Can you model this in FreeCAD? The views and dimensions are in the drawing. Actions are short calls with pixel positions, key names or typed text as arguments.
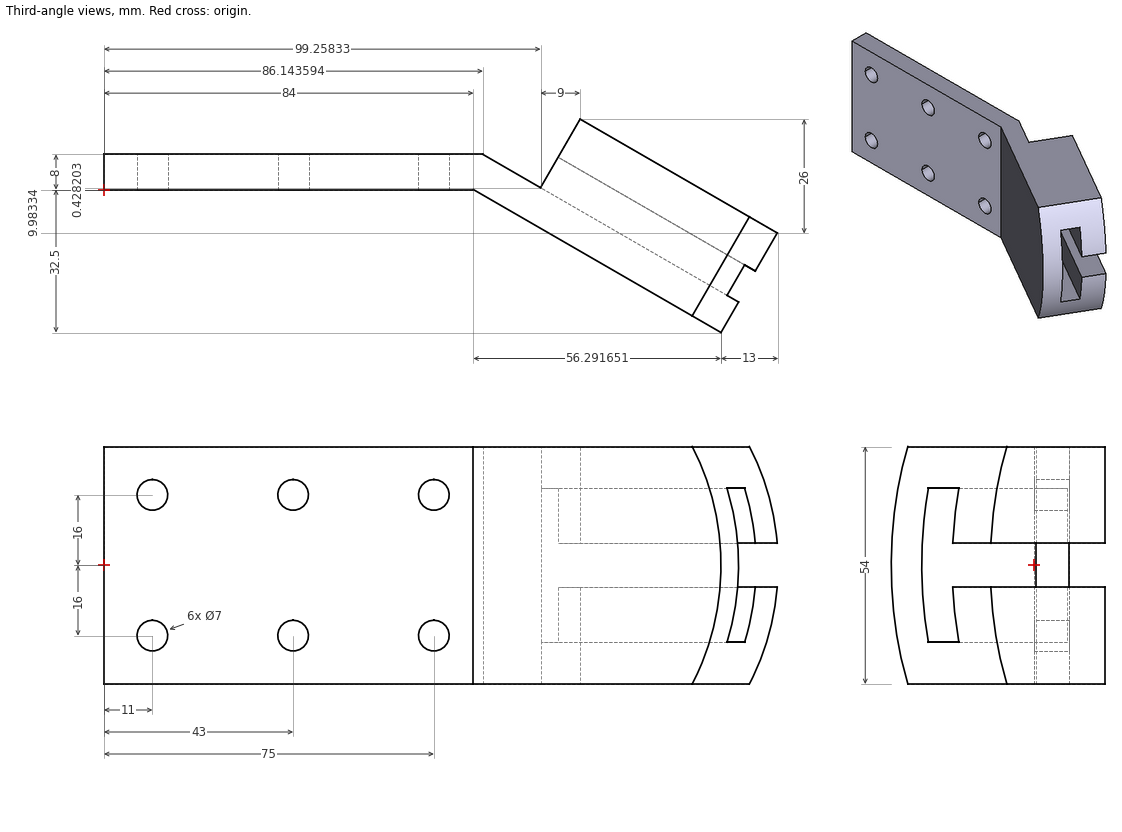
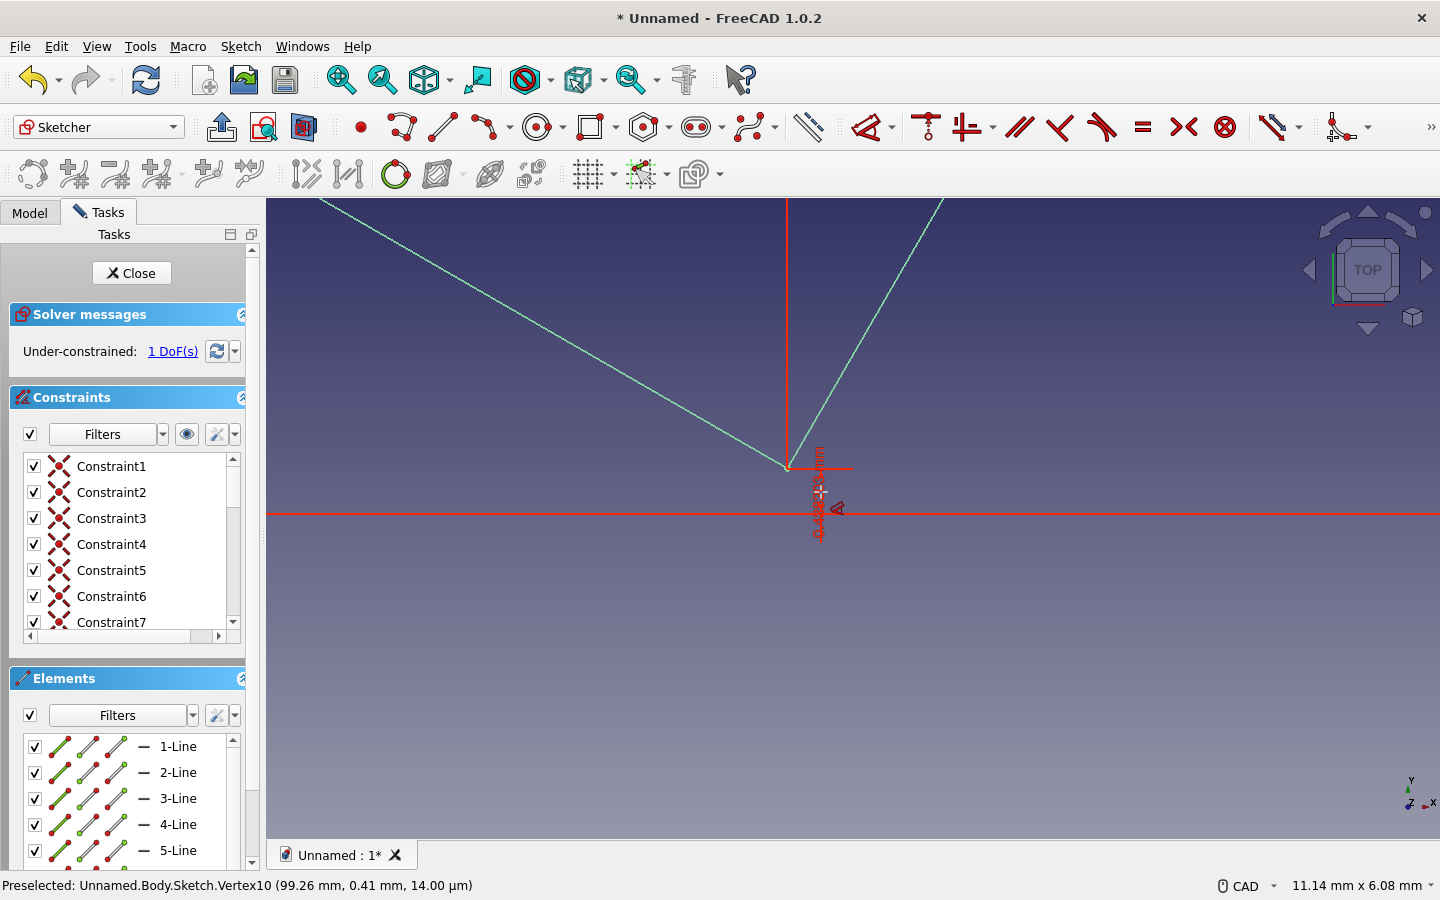
scroll(909, 473, down, 15)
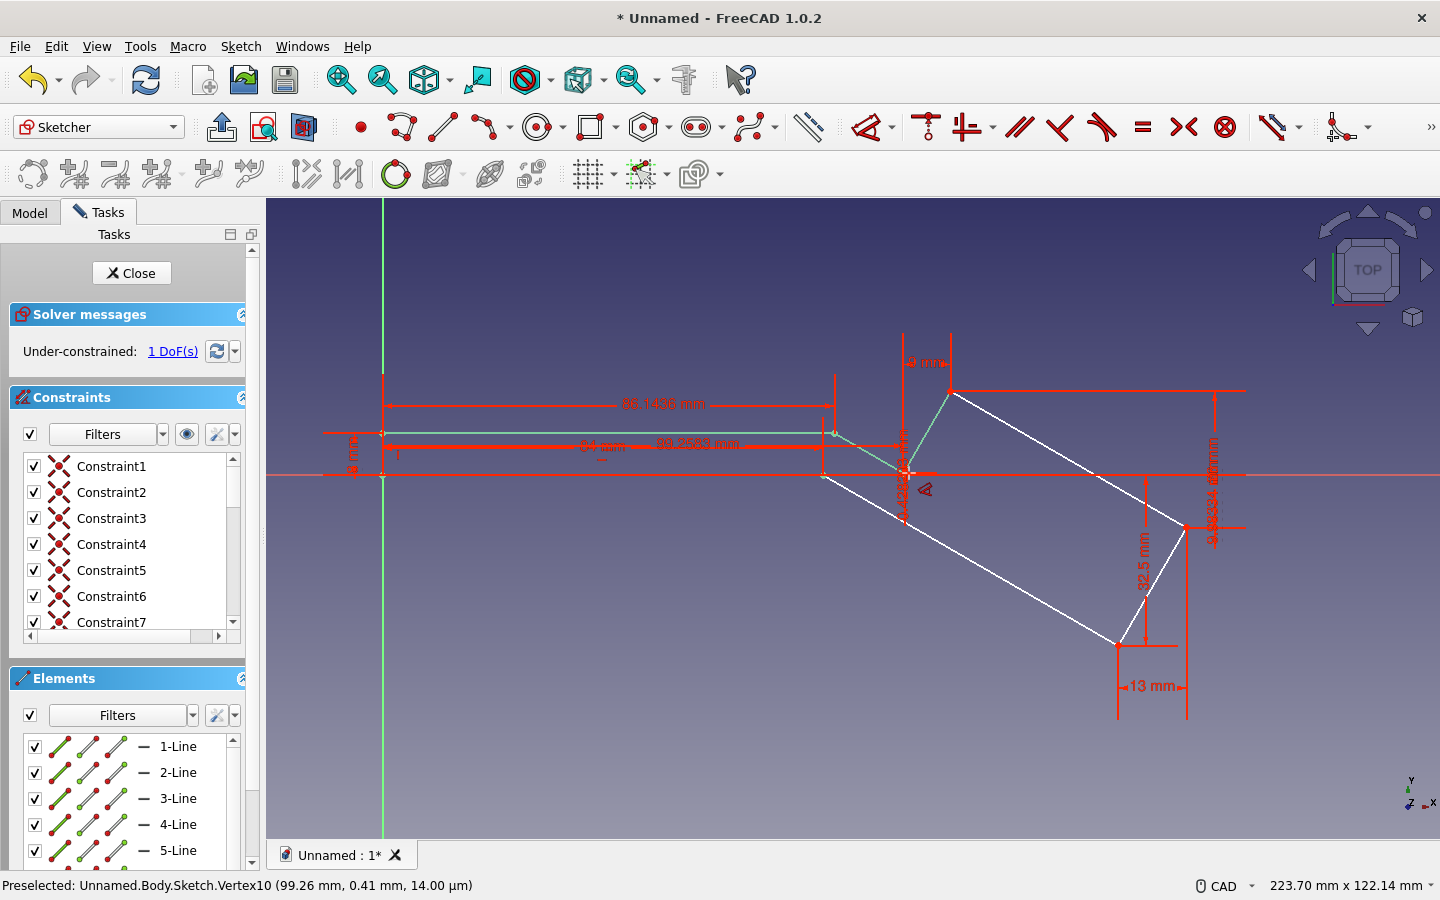
click(912, 527)
click(971, 680)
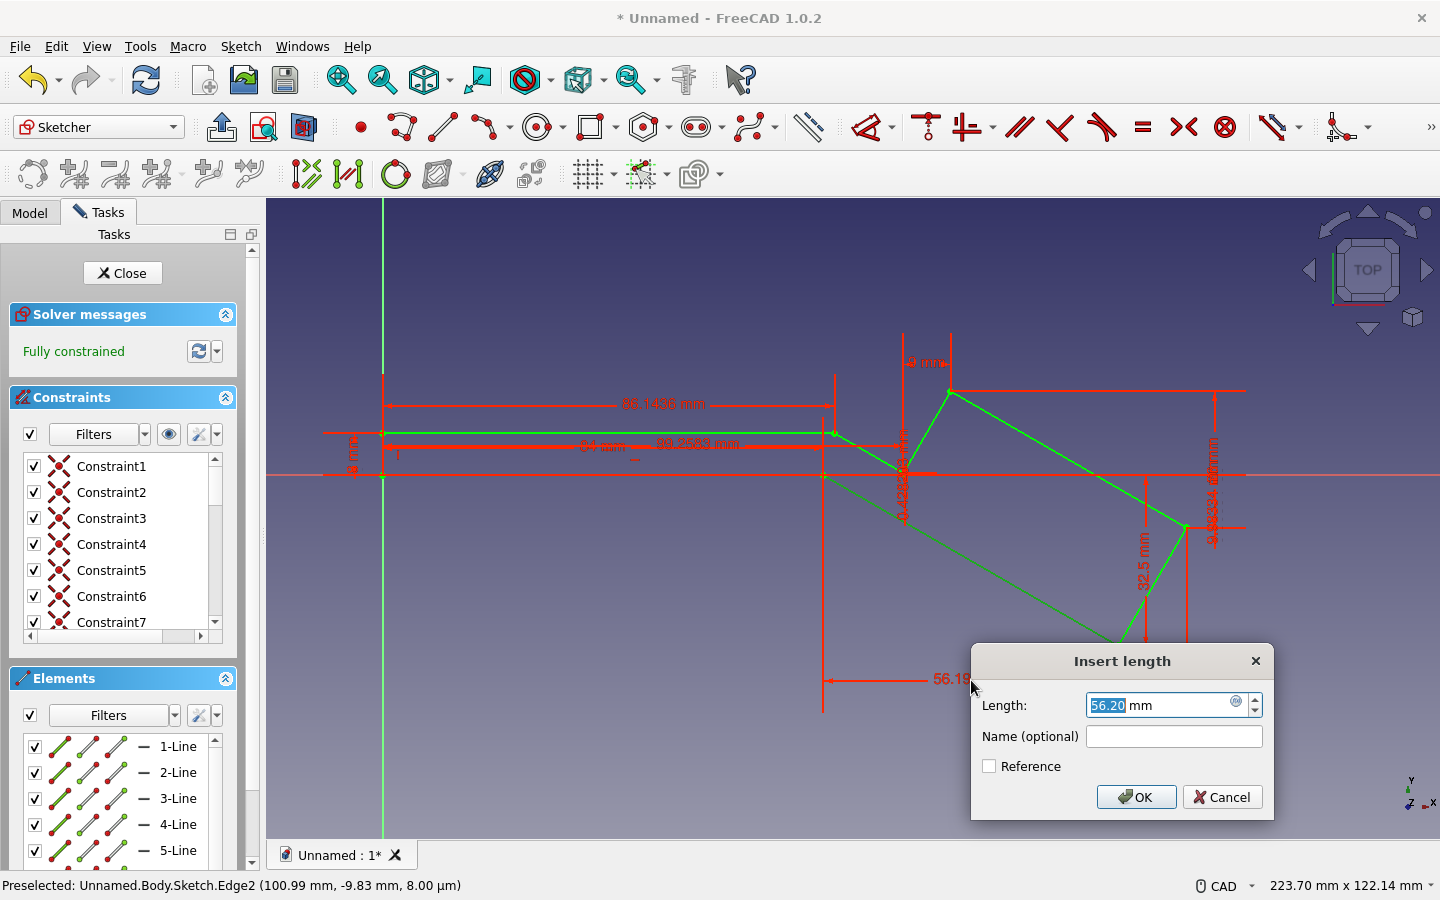
text(56.291651)
key(Return)
key(Escape)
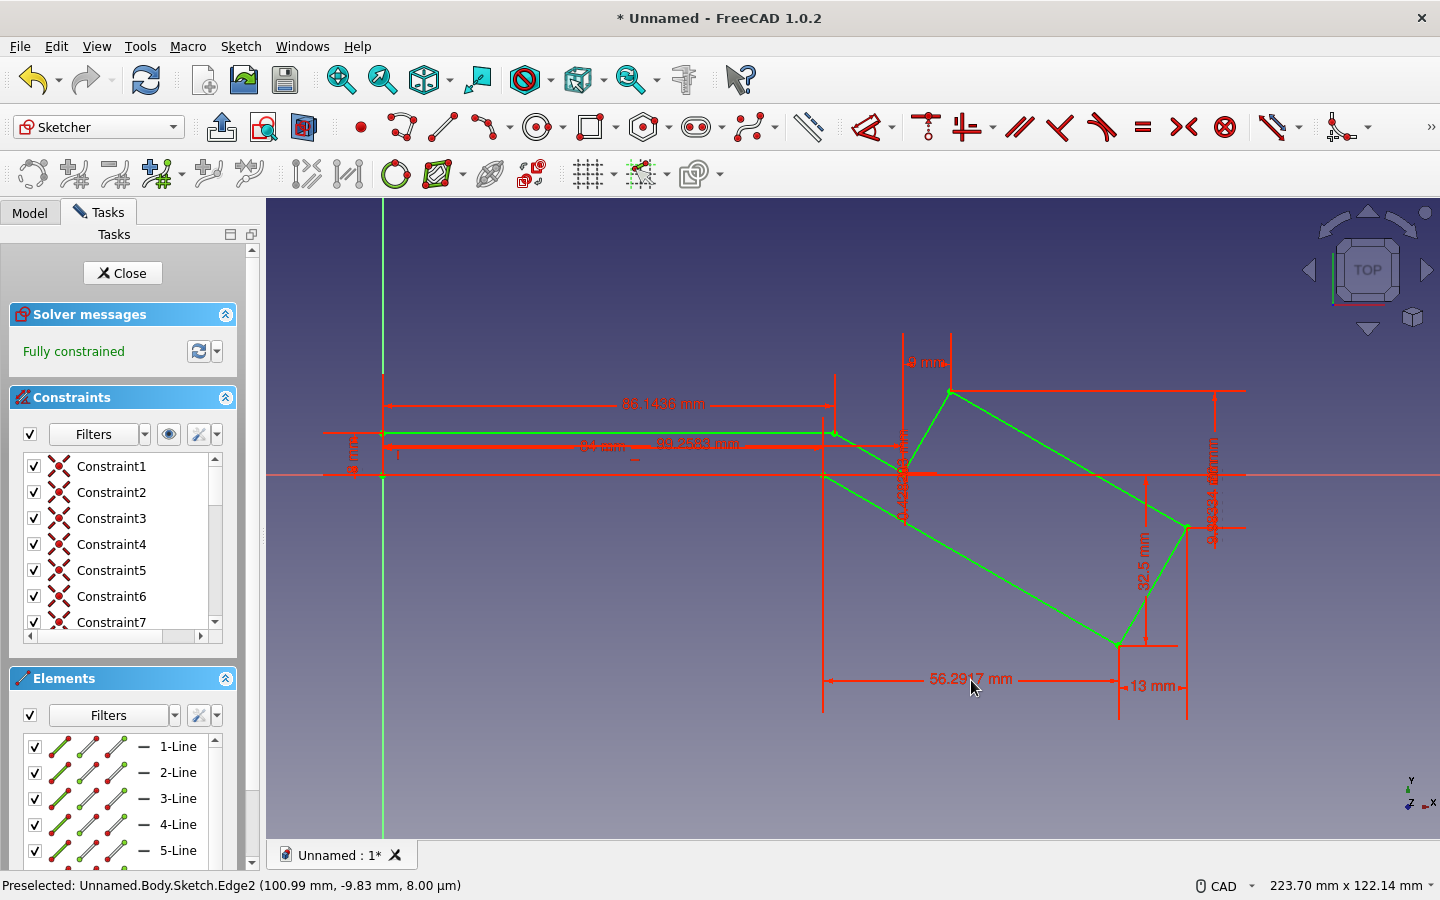
click(123, 273)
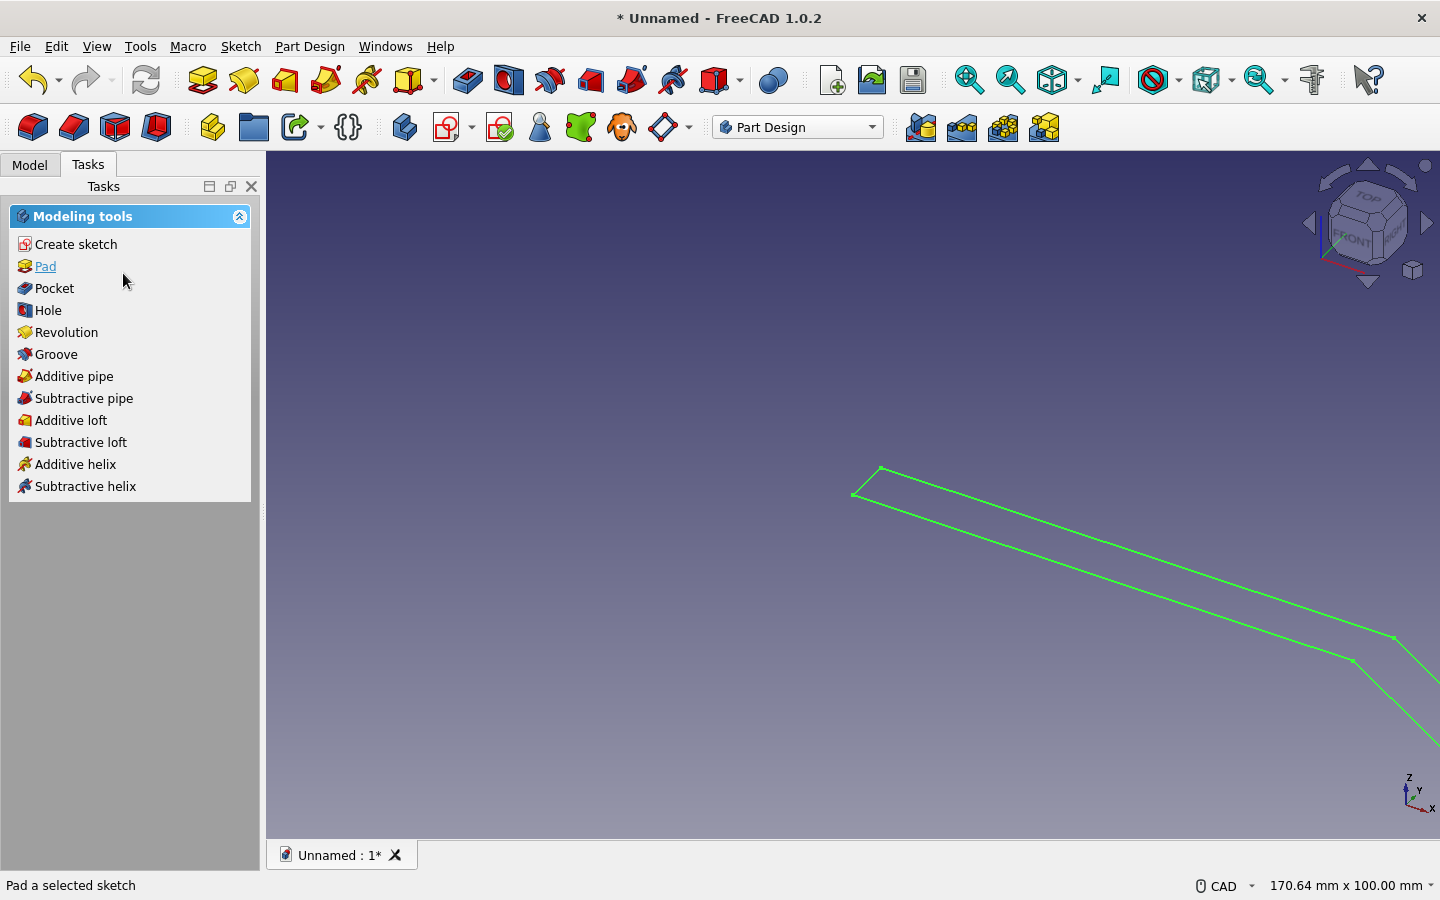
click(203, 80)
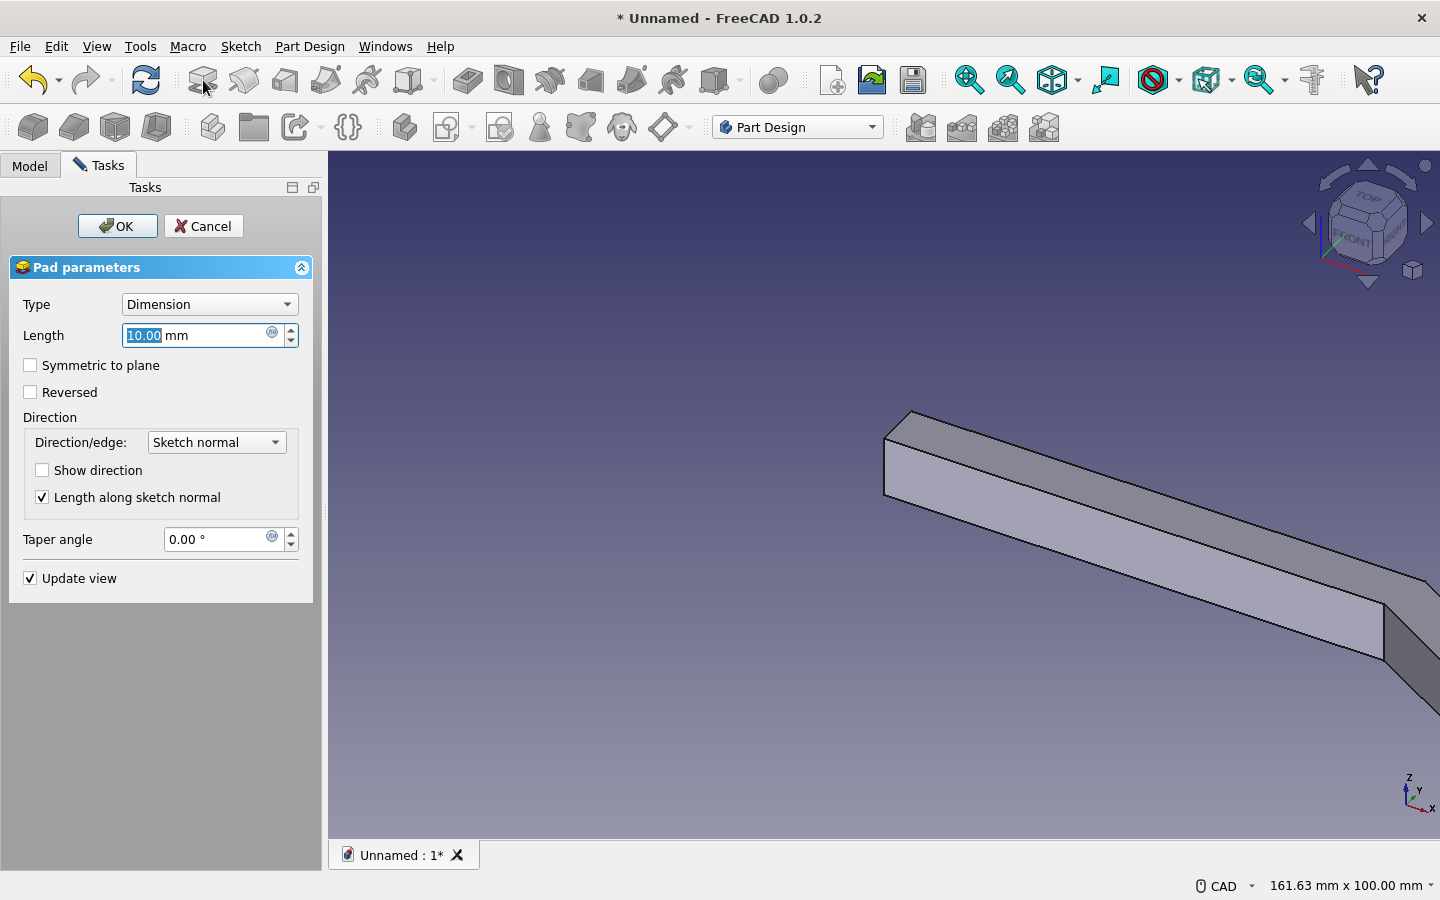
text(54)
key(Tab)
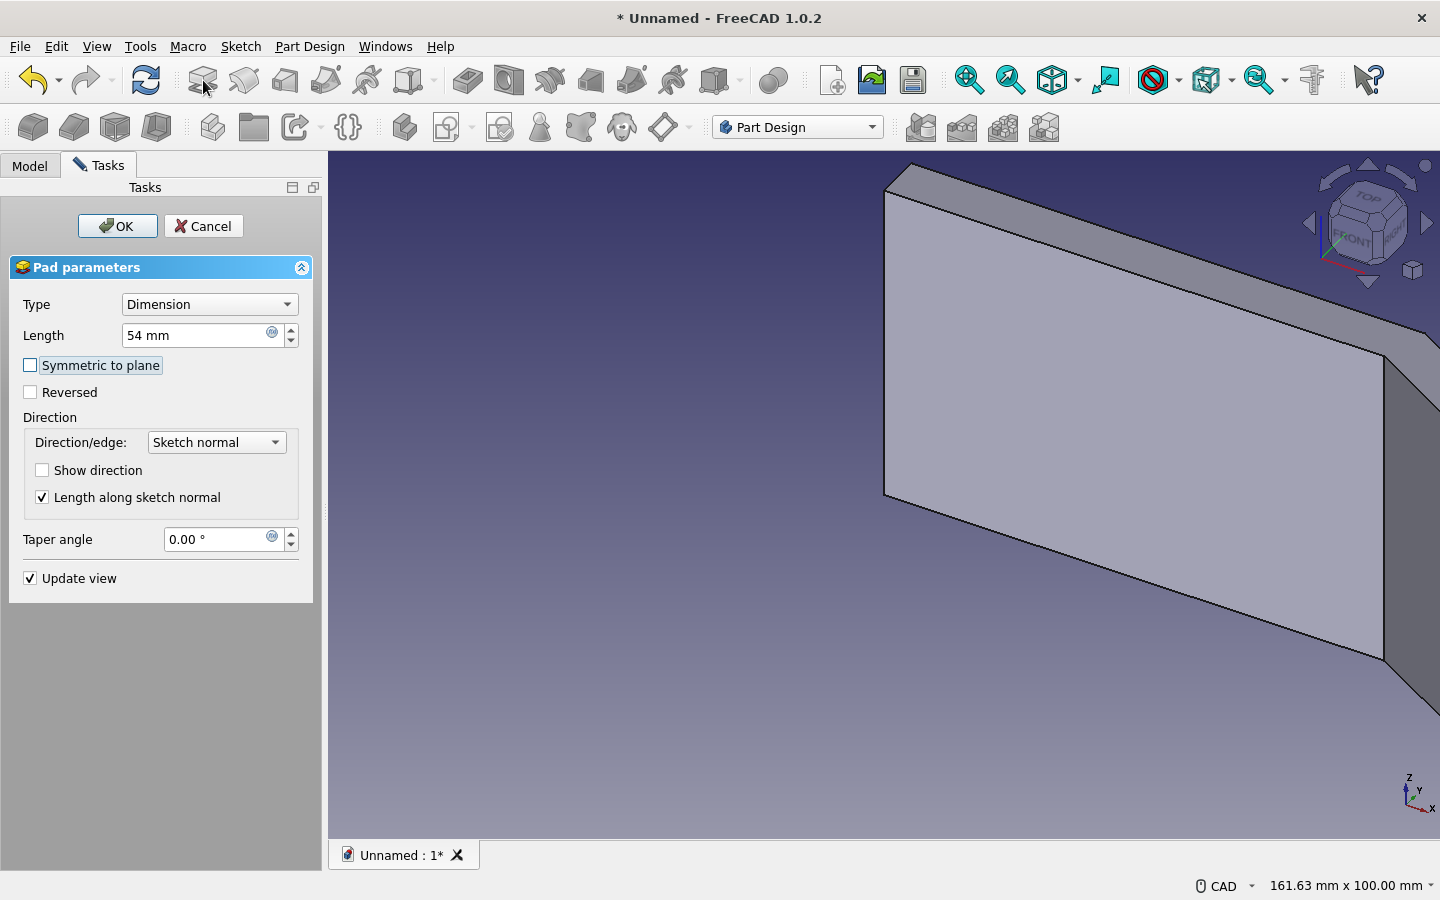
click(31, 365)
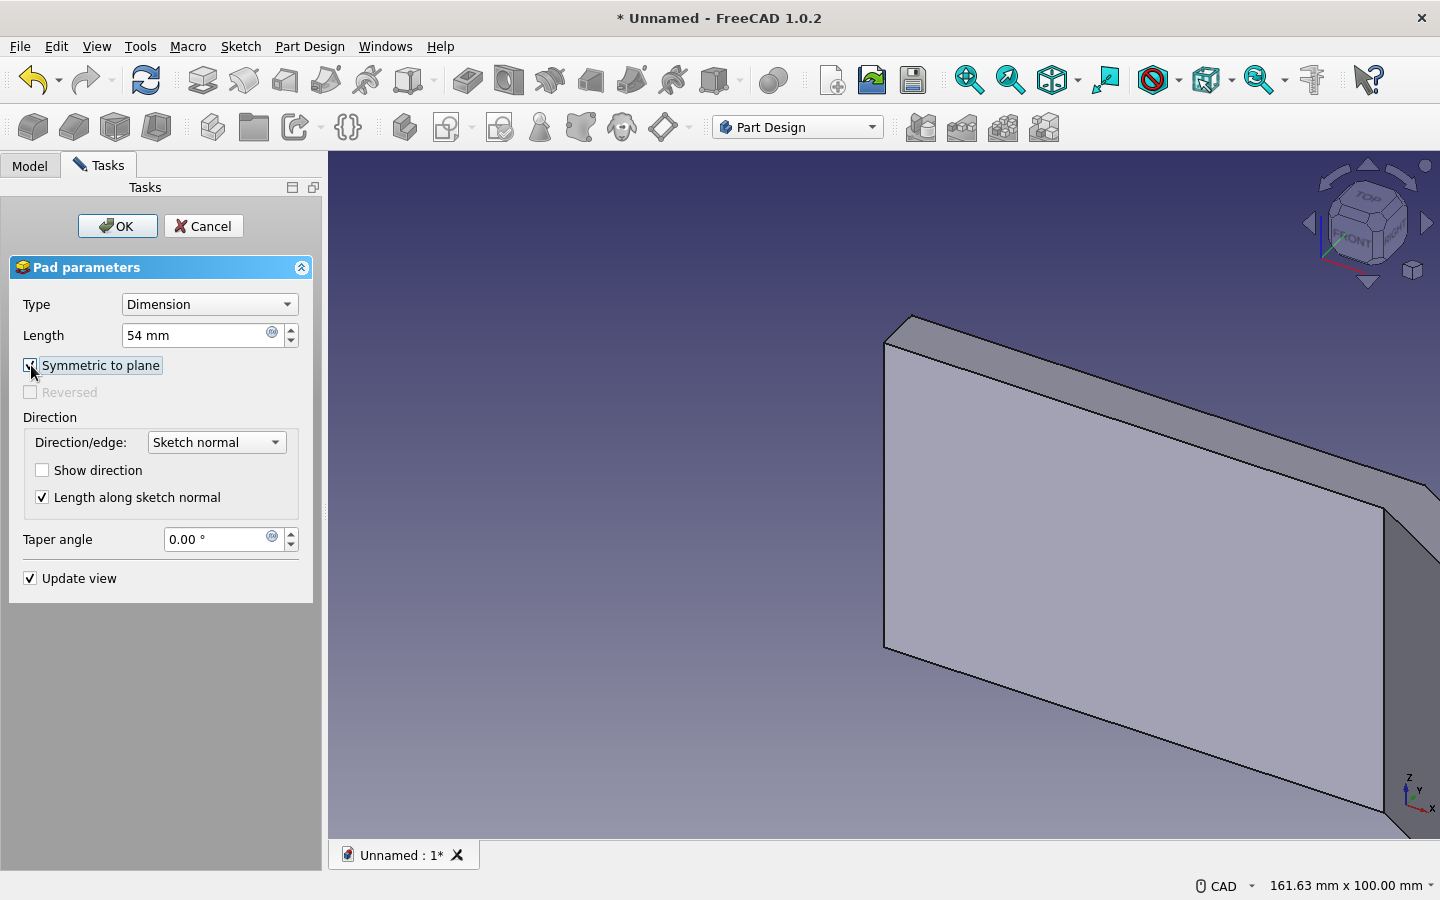
click(118, 226)